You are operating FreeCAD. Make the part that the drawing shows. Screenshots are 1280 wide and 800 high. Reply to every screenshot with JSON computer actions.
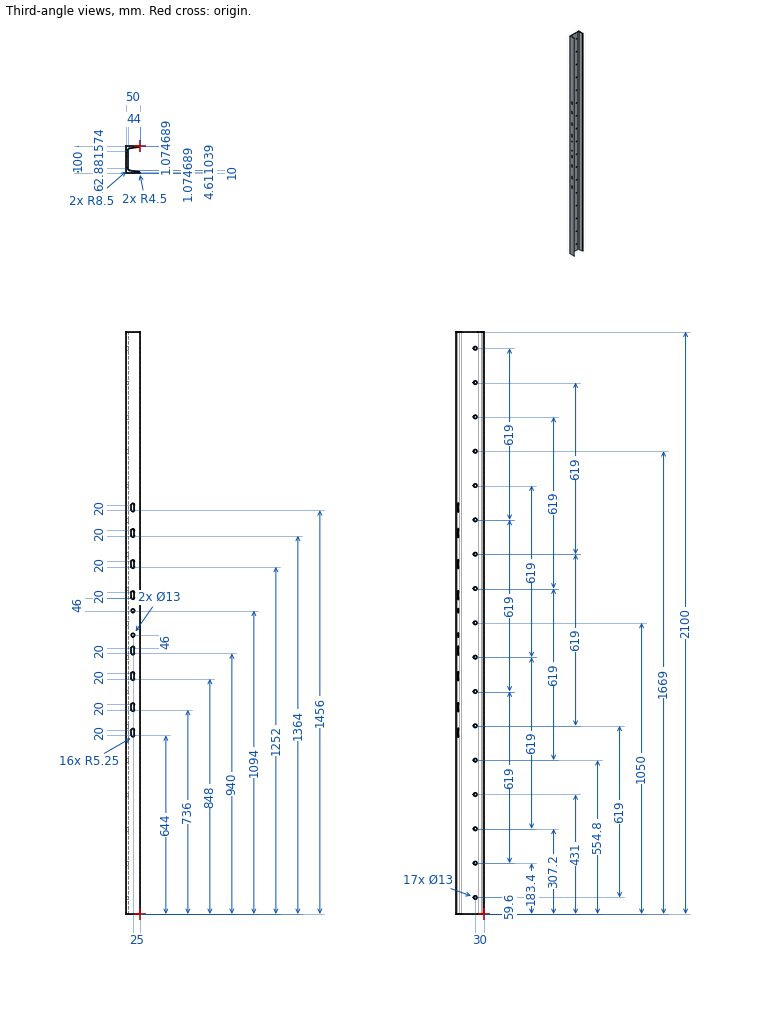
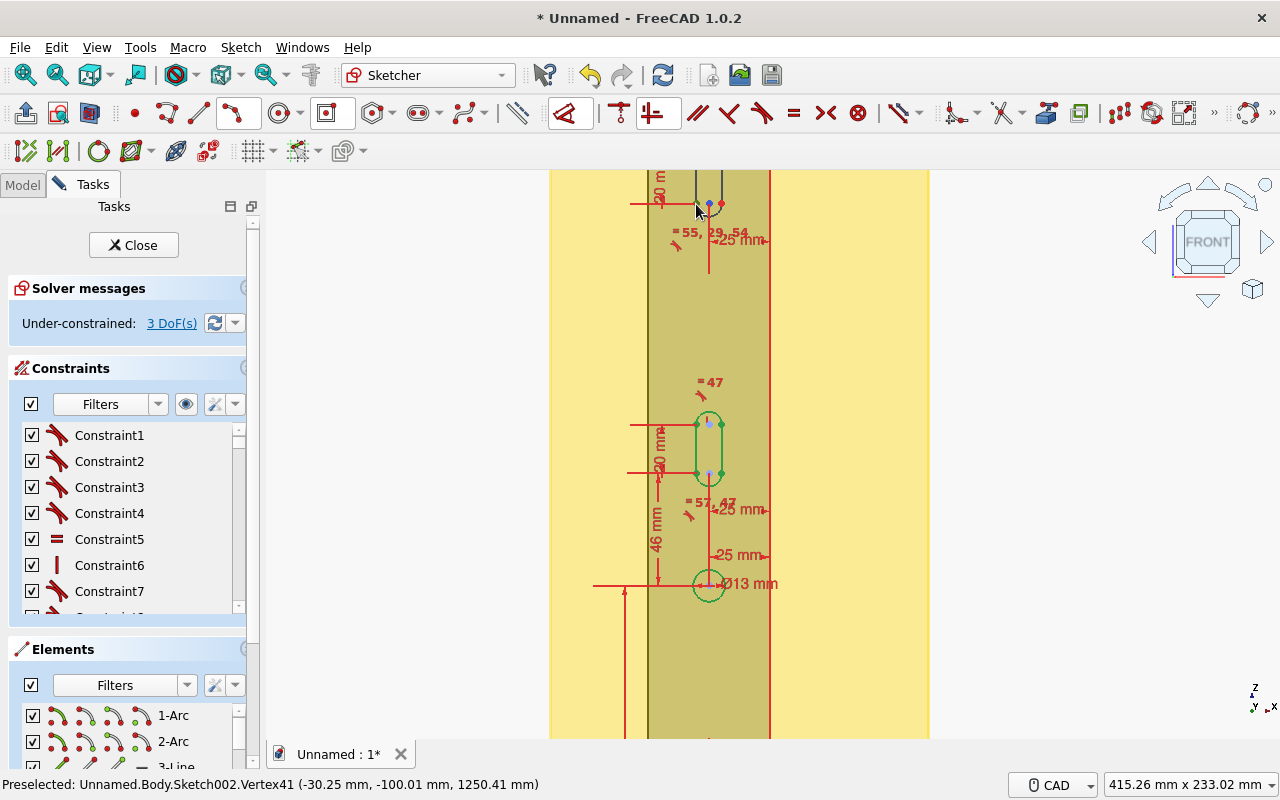
{"action": "left_click", "coordinate": [588, 114]}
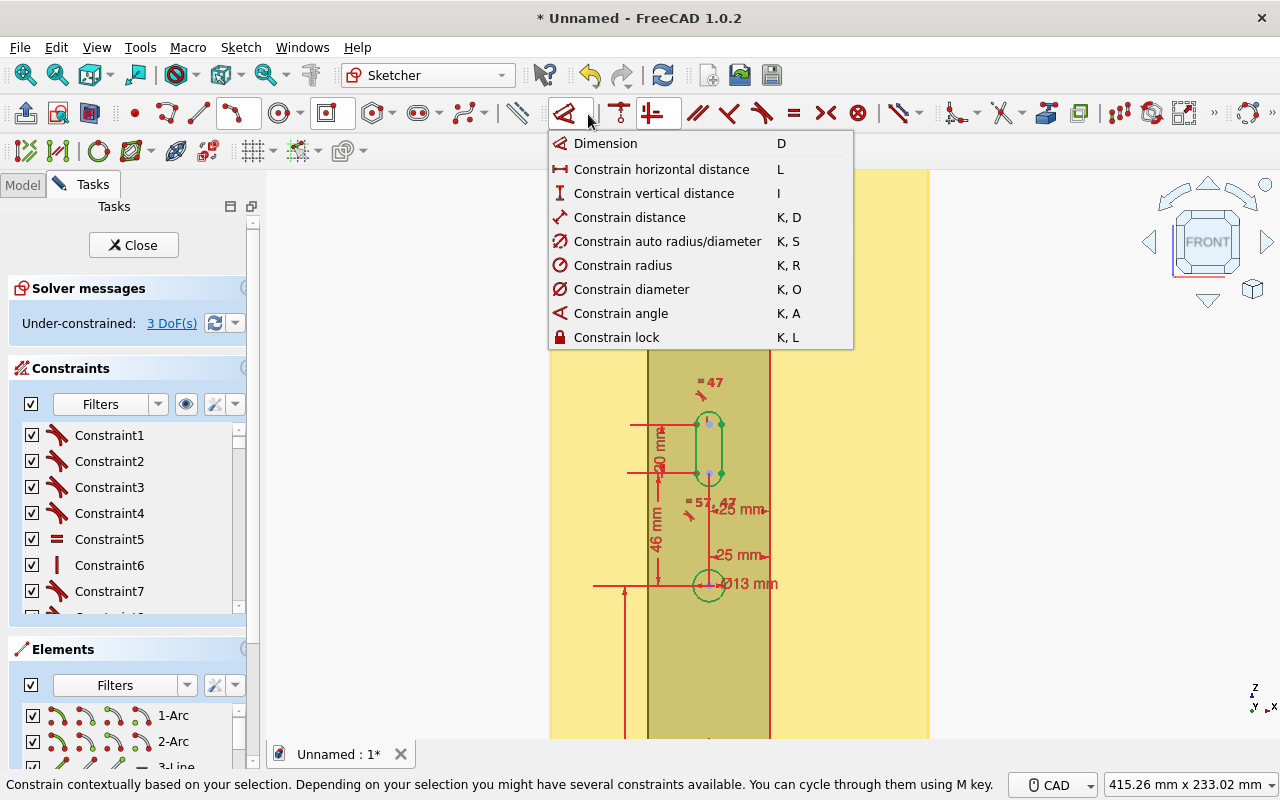
{"action": "left_click", "coordinate": [701, 193]}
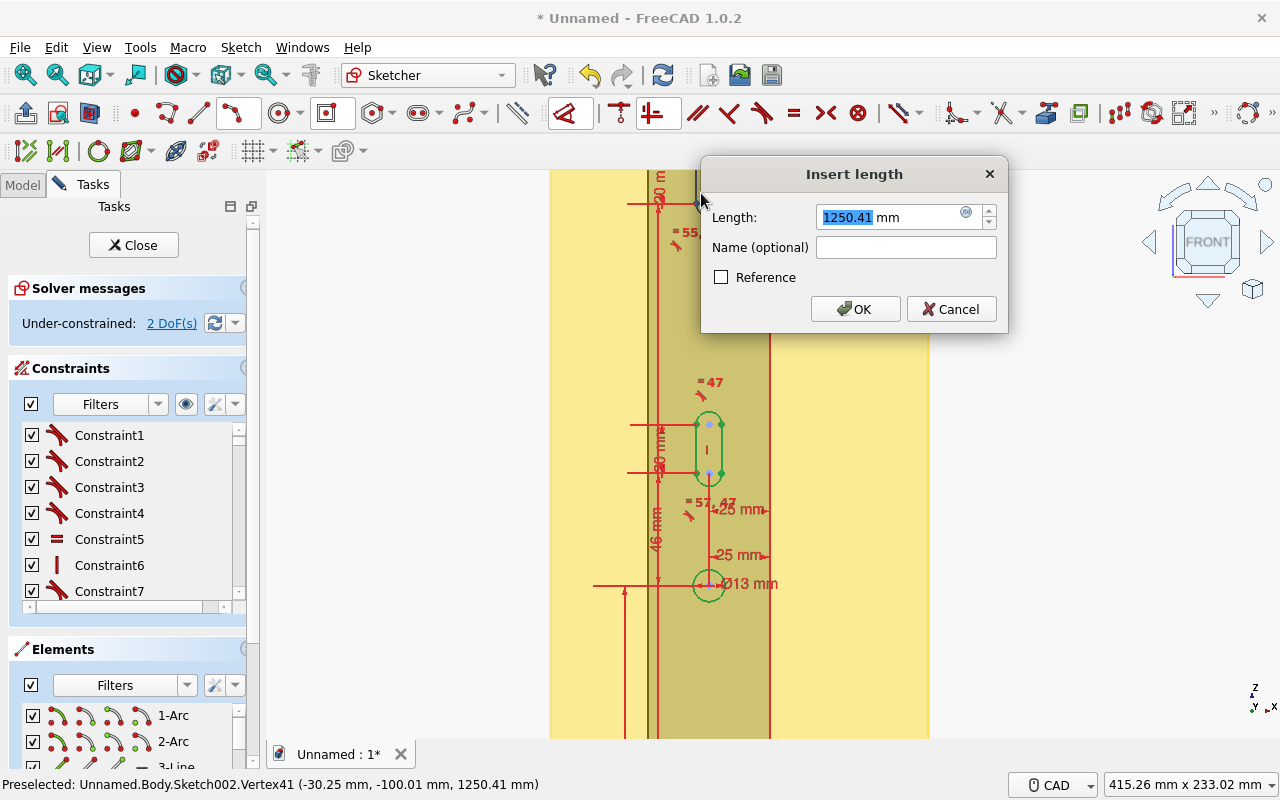
{"action": "type", "text": "1252"}
{"action": "key", "text": "Return"}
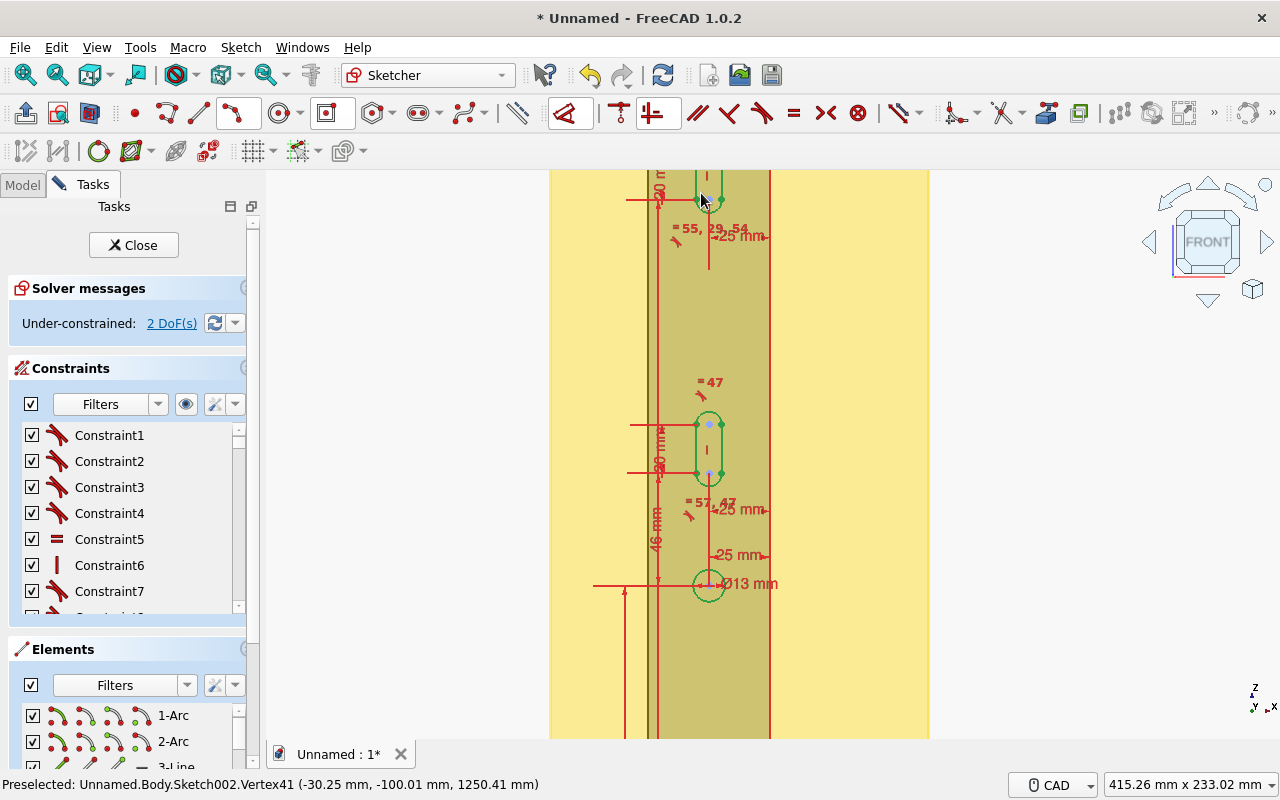
{"action": "scroll", "coordinate": [702, 355], "scroll_direction": "down", "scroll_amount": 12}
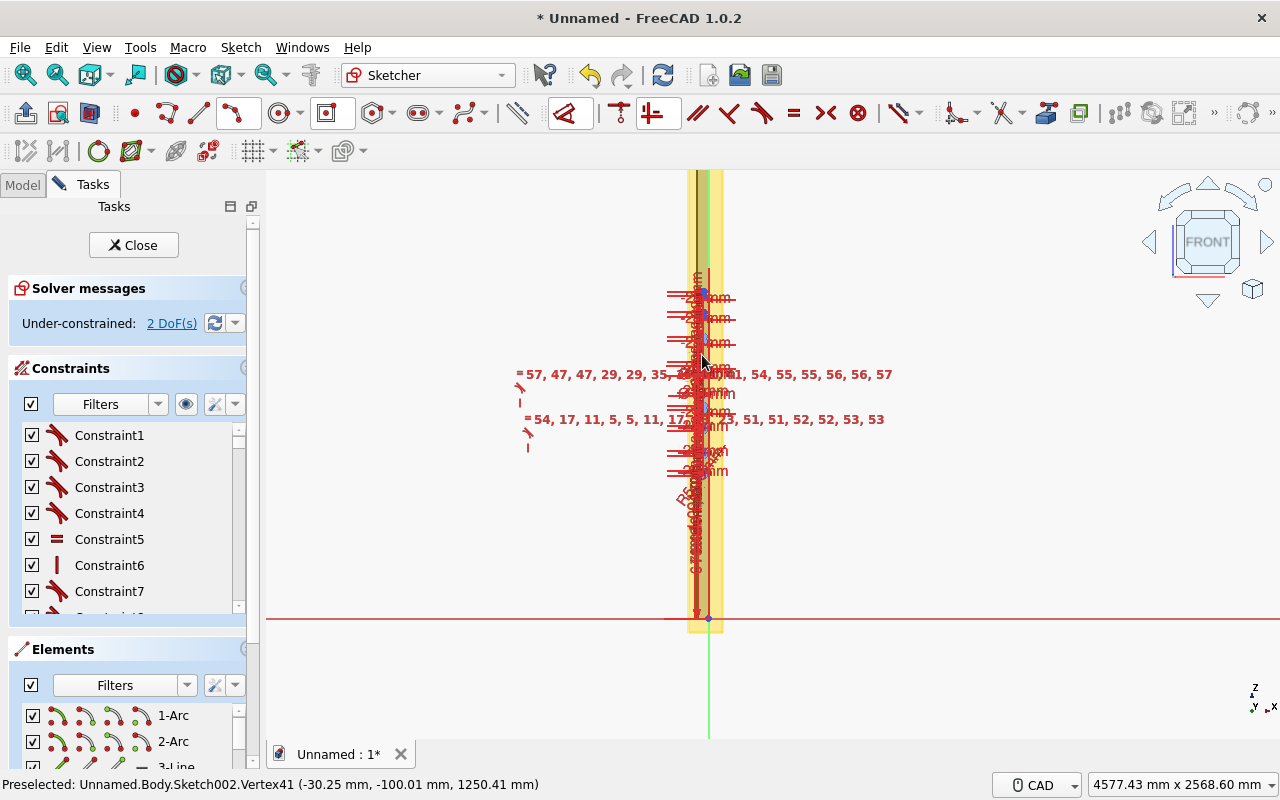
{"action": "scroll", "coordinate": [702, 296], "scroll_direction": "up", "scroll_amount": 12}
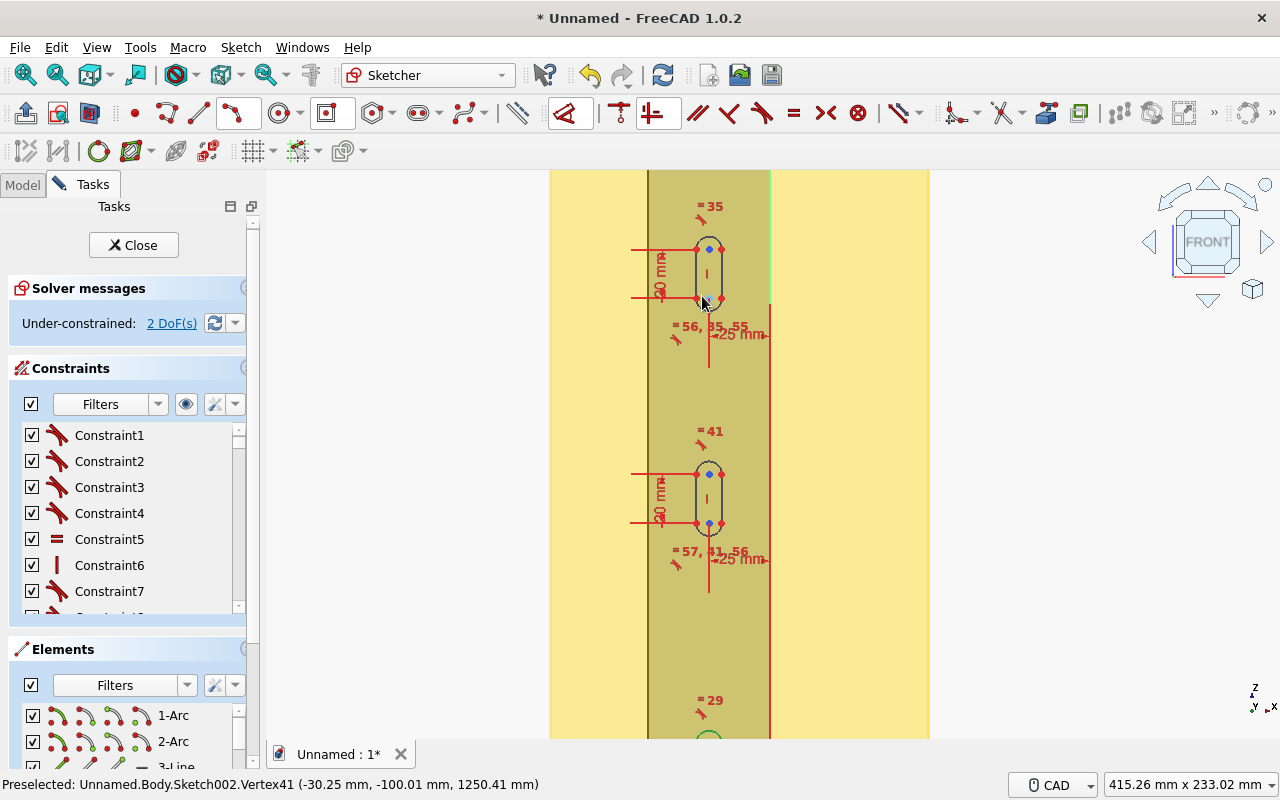
{"action": "left_click", "coordinate": [696, 298]}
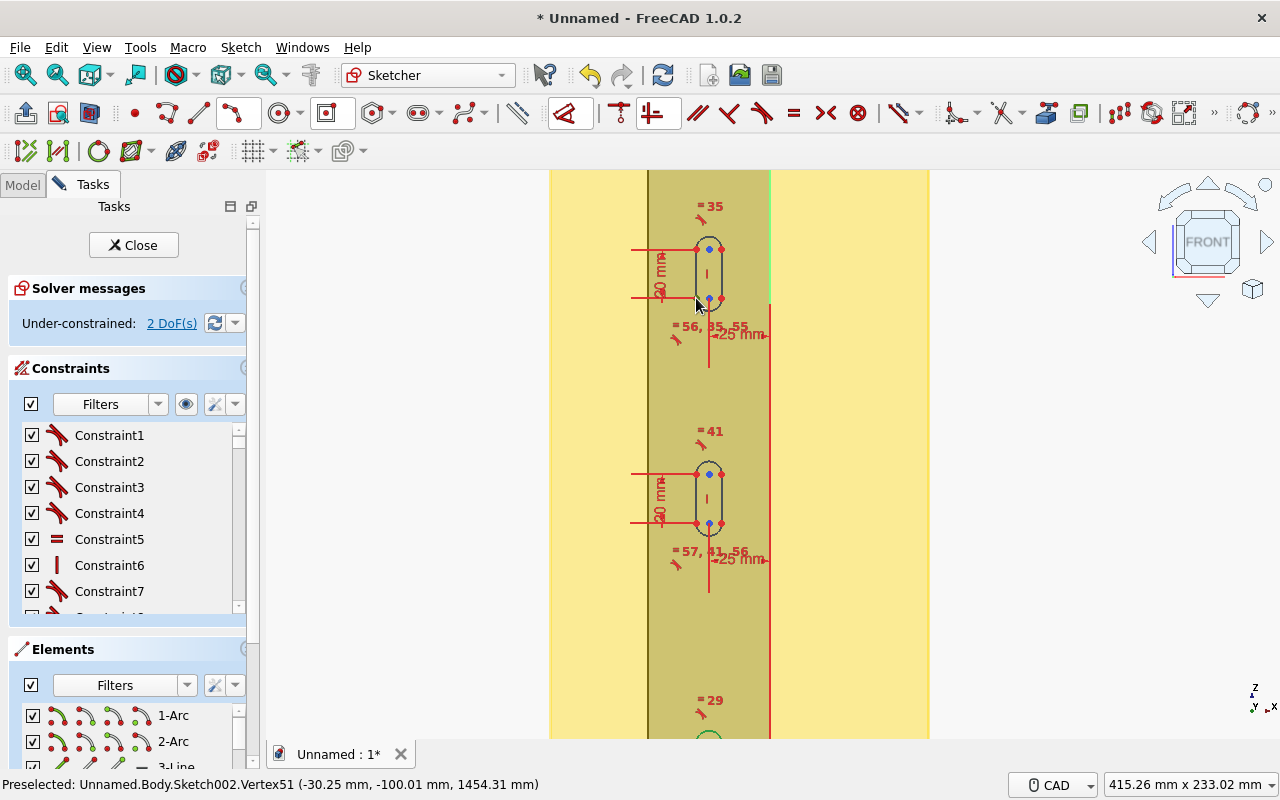
{"action": "left_click", "coordinate": [588, 114]}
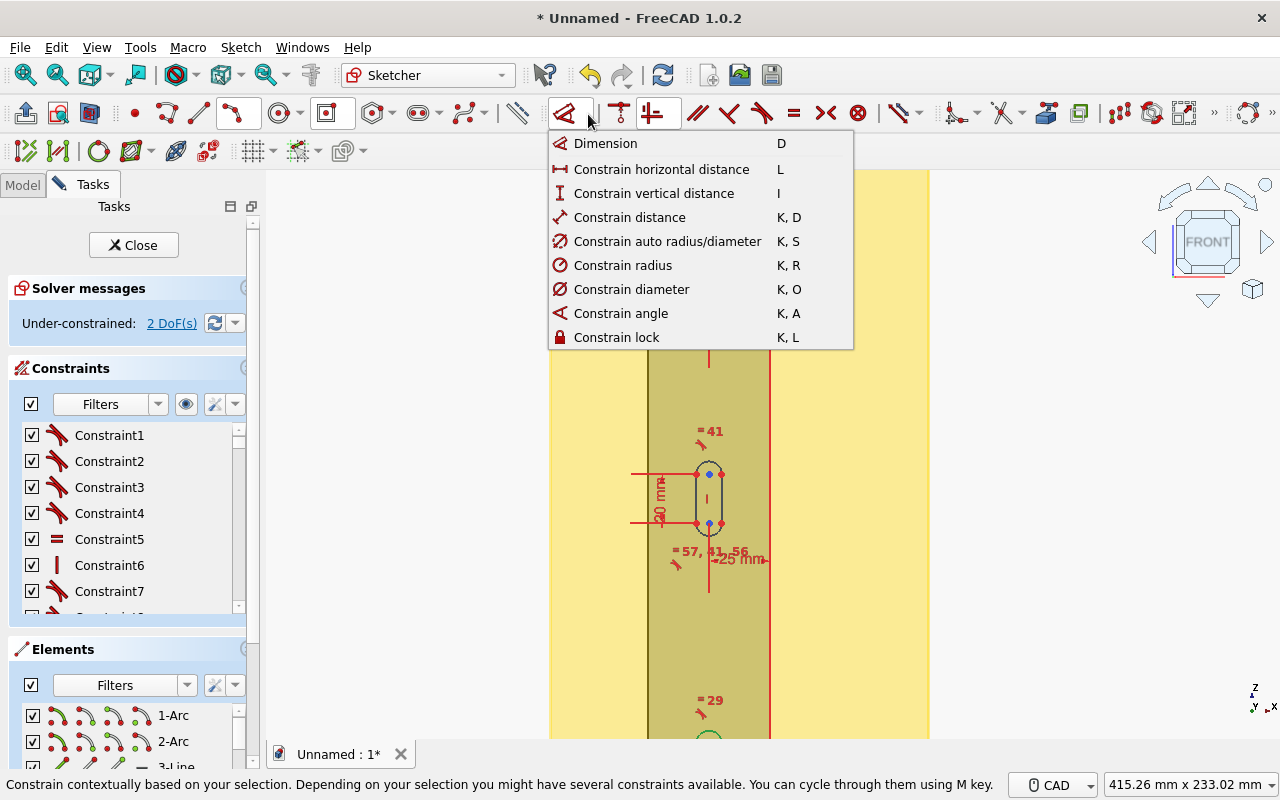
{"action": "left_click", "coordinate": [701, 193]}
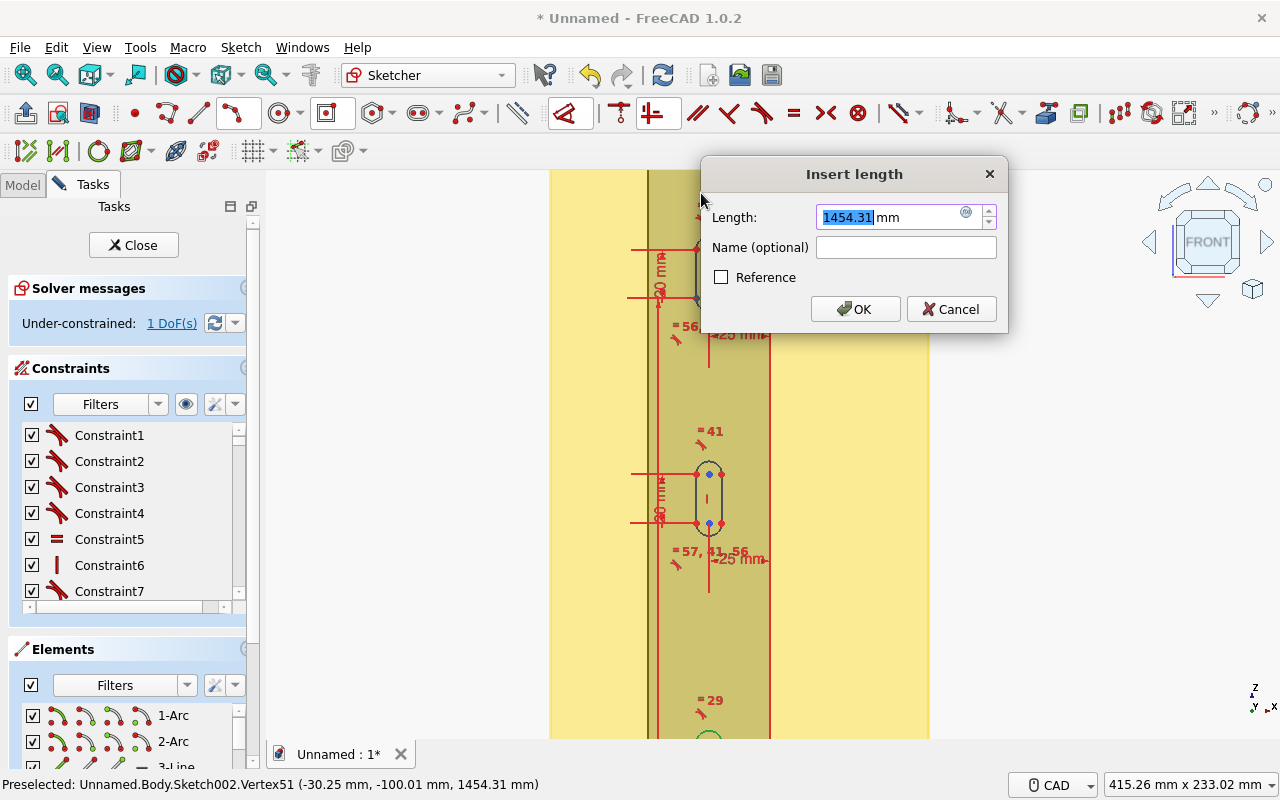
{"action": "type", "text": "1456"}
{"action": "key", "text": "Return"}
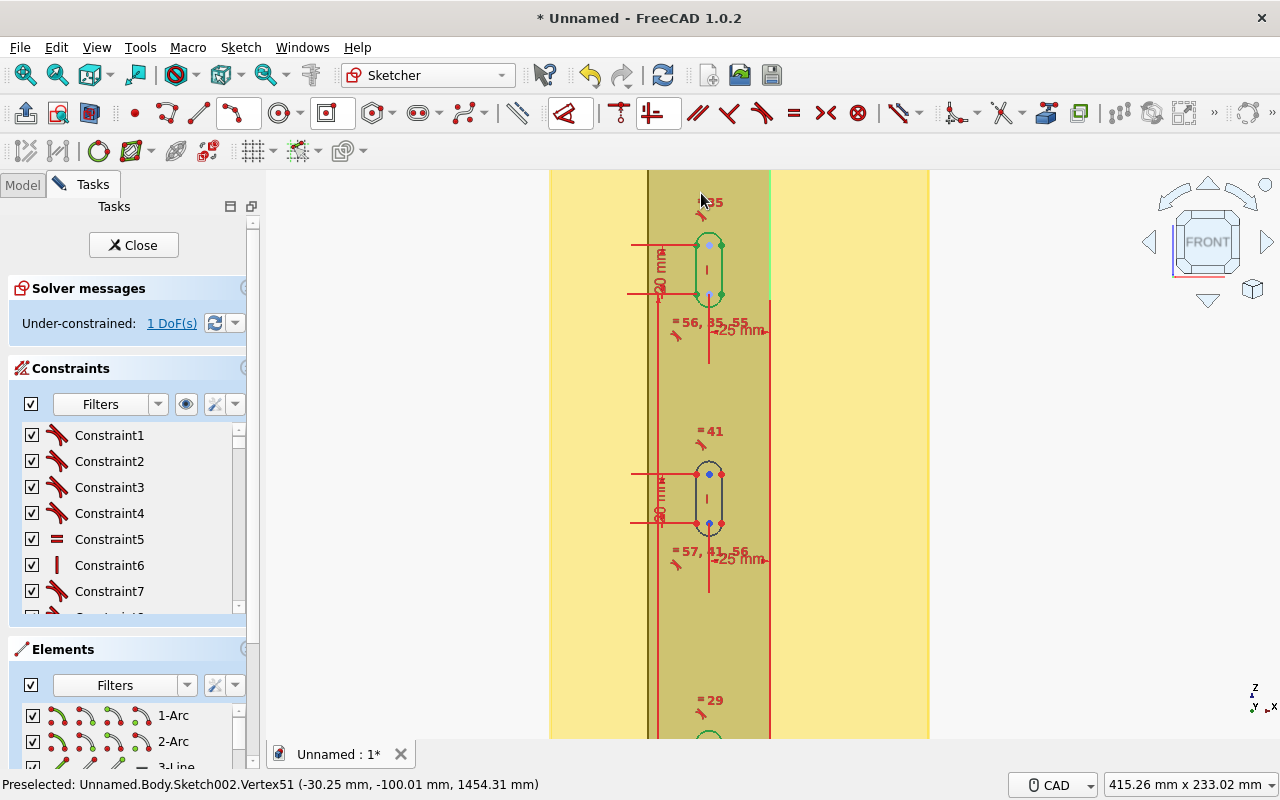
{"action": "left_click", "coordinate": [696, 523]}